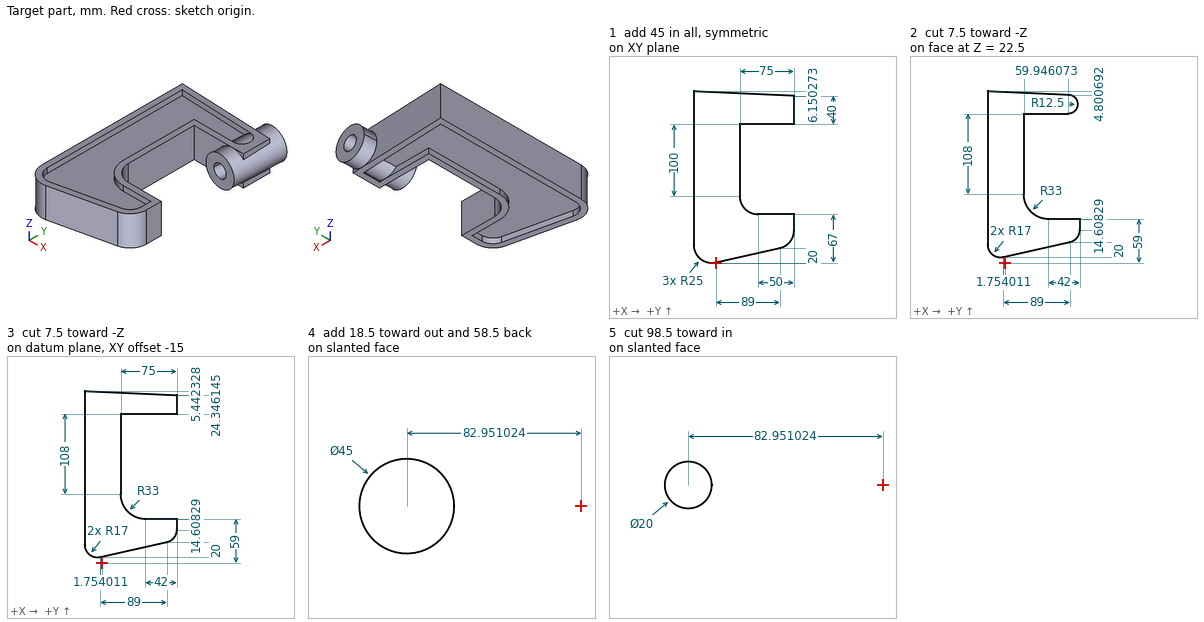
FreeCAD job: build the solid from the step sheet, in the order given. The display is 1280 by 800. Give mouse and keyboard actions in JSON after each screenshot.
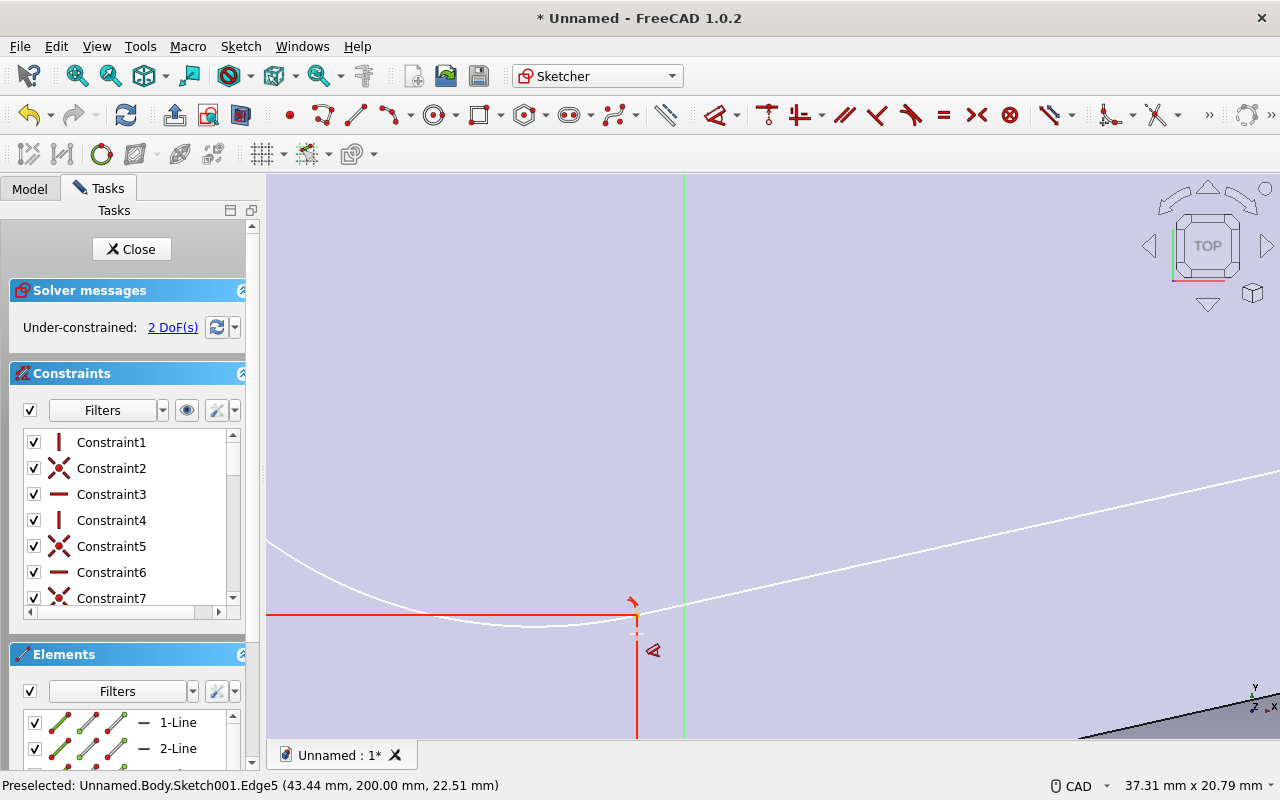
{"action": "left_click", "coordinate": [637, 615]}
{"action": "left_click", "coordinate": [660, 581]}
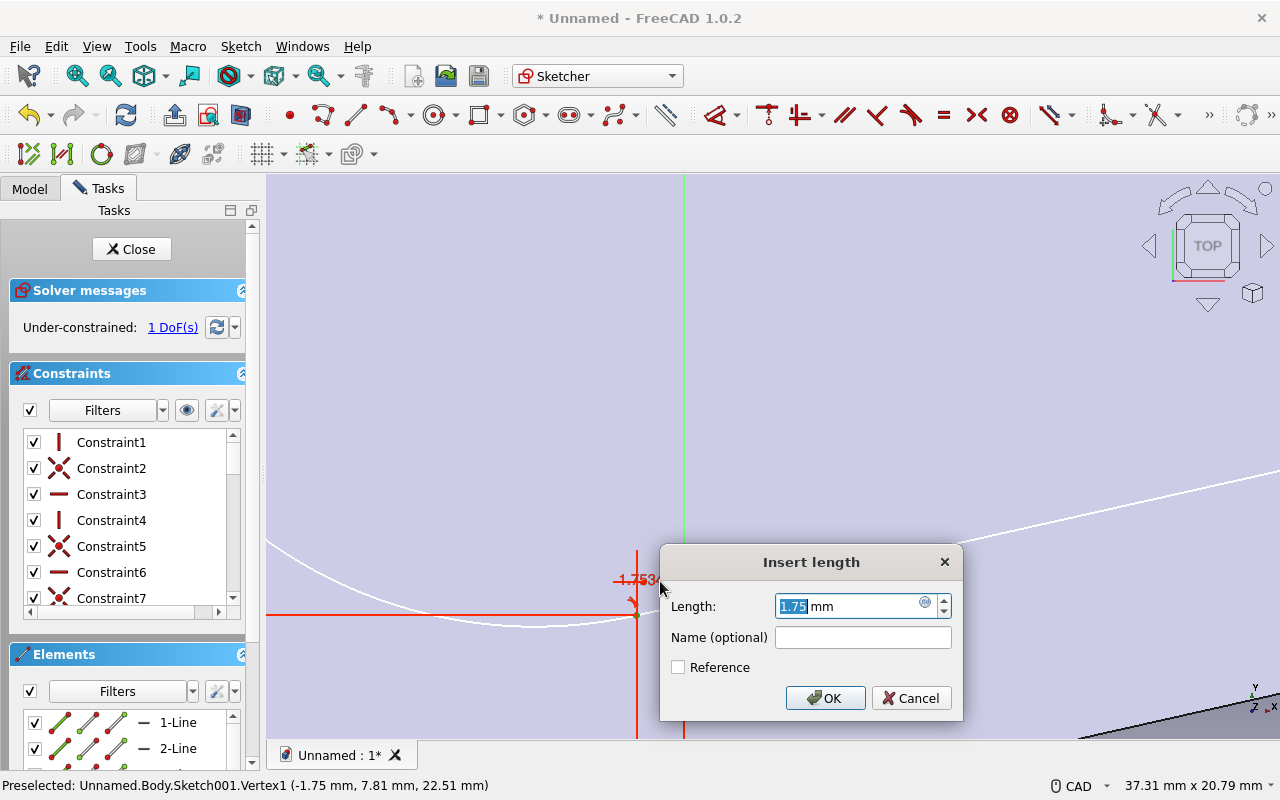
{"action": "type", "text": "1.754011"}
{"action": "key", "text": "Return"}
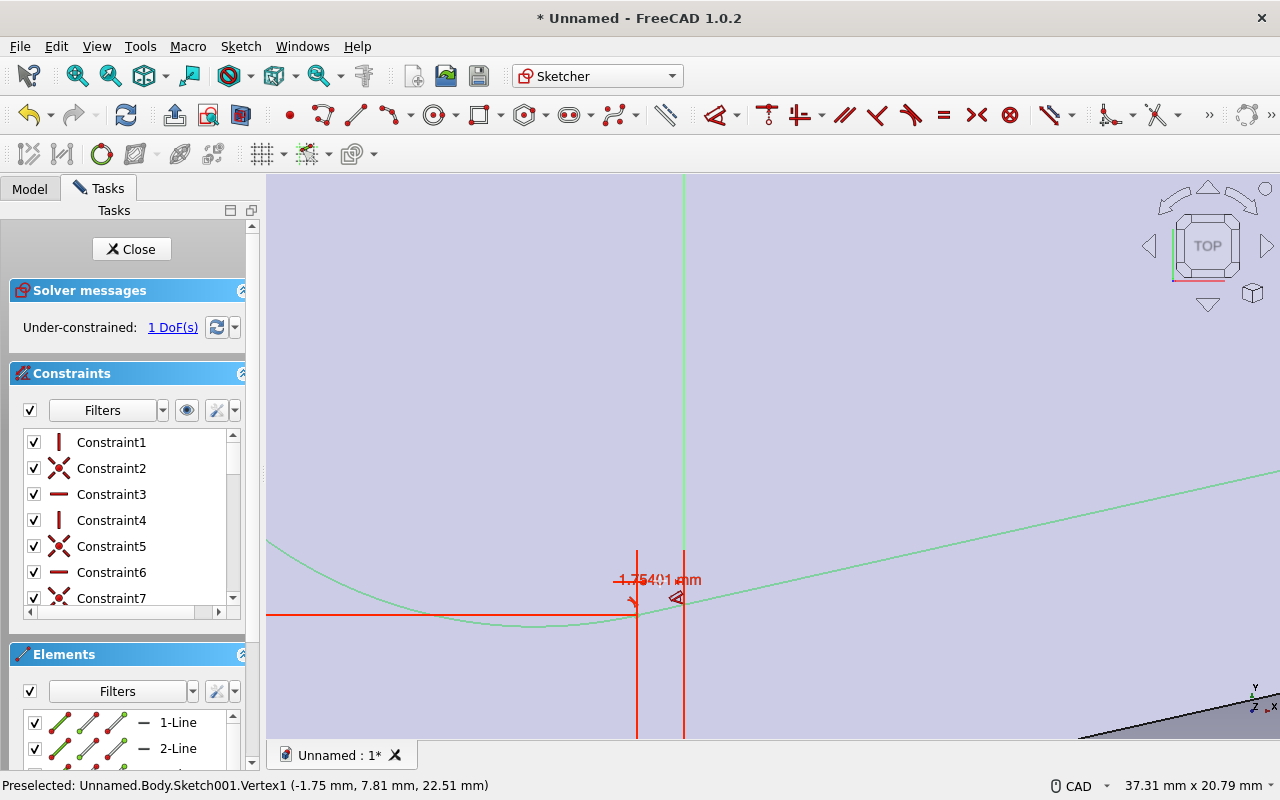
{"action": "scroll", "coordinate": [637, 635], "scroll_direction": "down", "scroll_amount": 14}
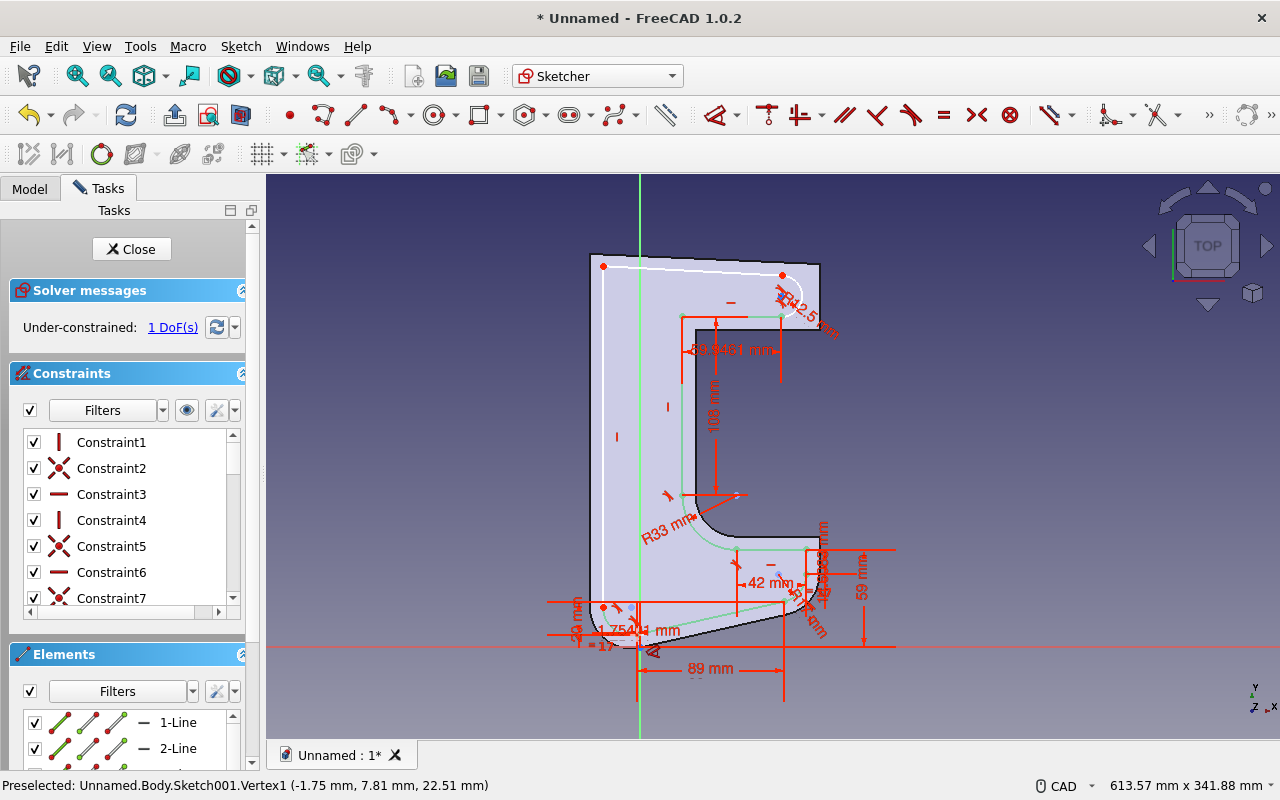
{"action": "scroll", "coordinate": [729, 273], "scroll_direction": "up", "scroll_amount": 9}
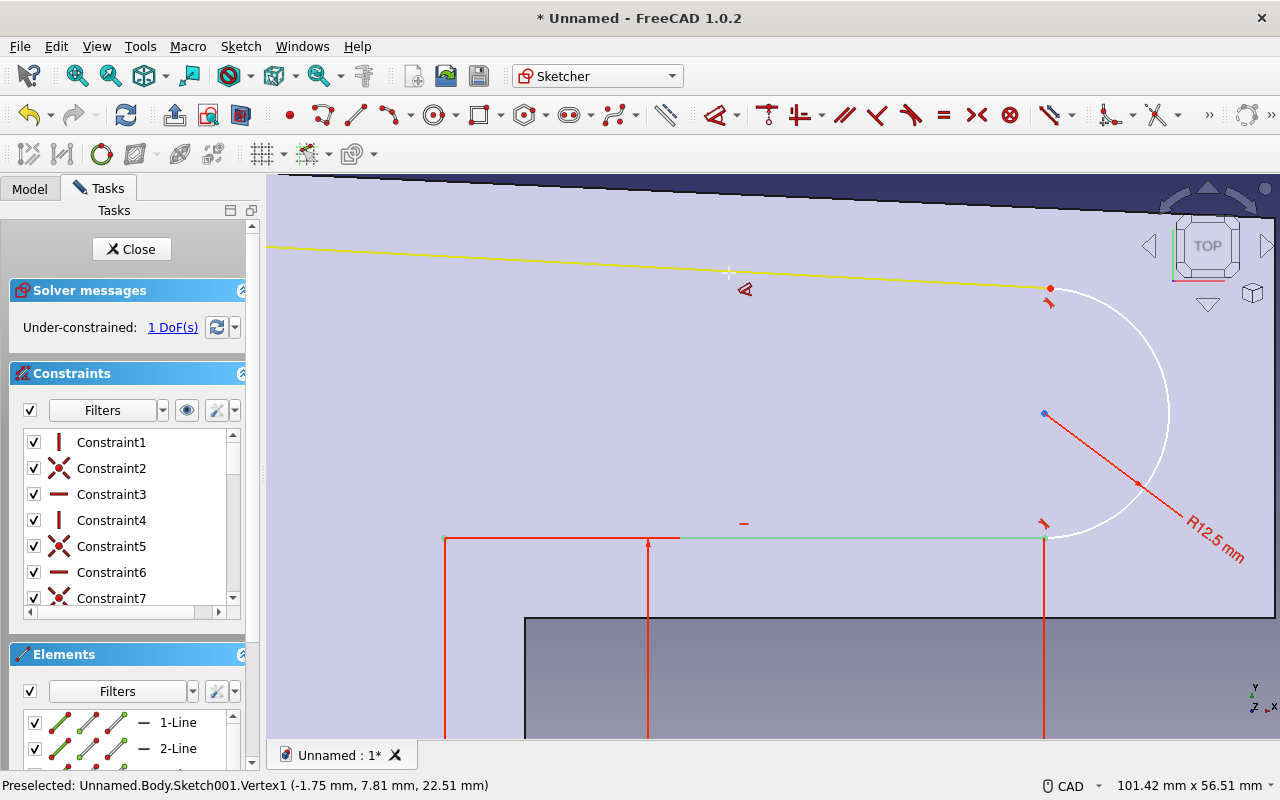
{"action": "left_click", "coordinate": [725, 271]}
{"action": "left_click", "coordinate": [1085, 260]}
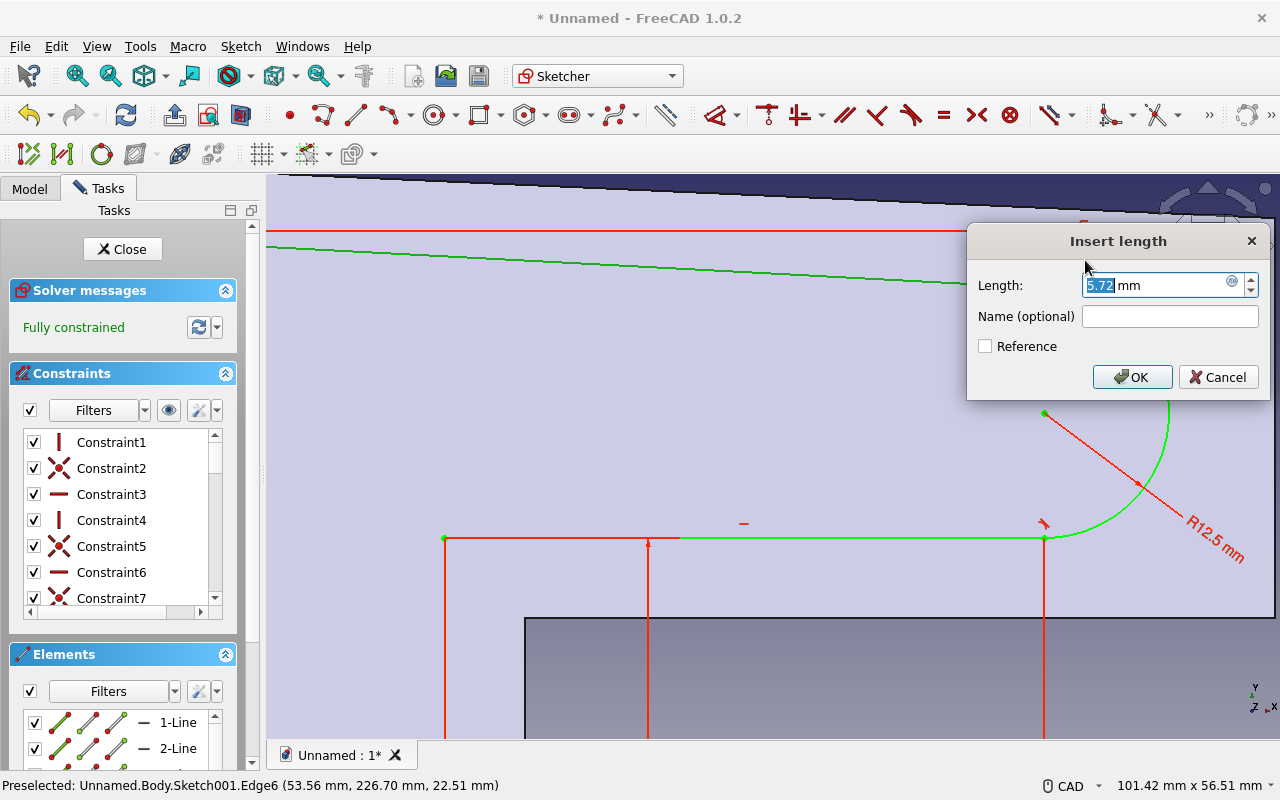
{"action": "type", "text": "4.800692"}
{"action": "key", "text": "Return"}
{"action": "key", "text": "Escape"}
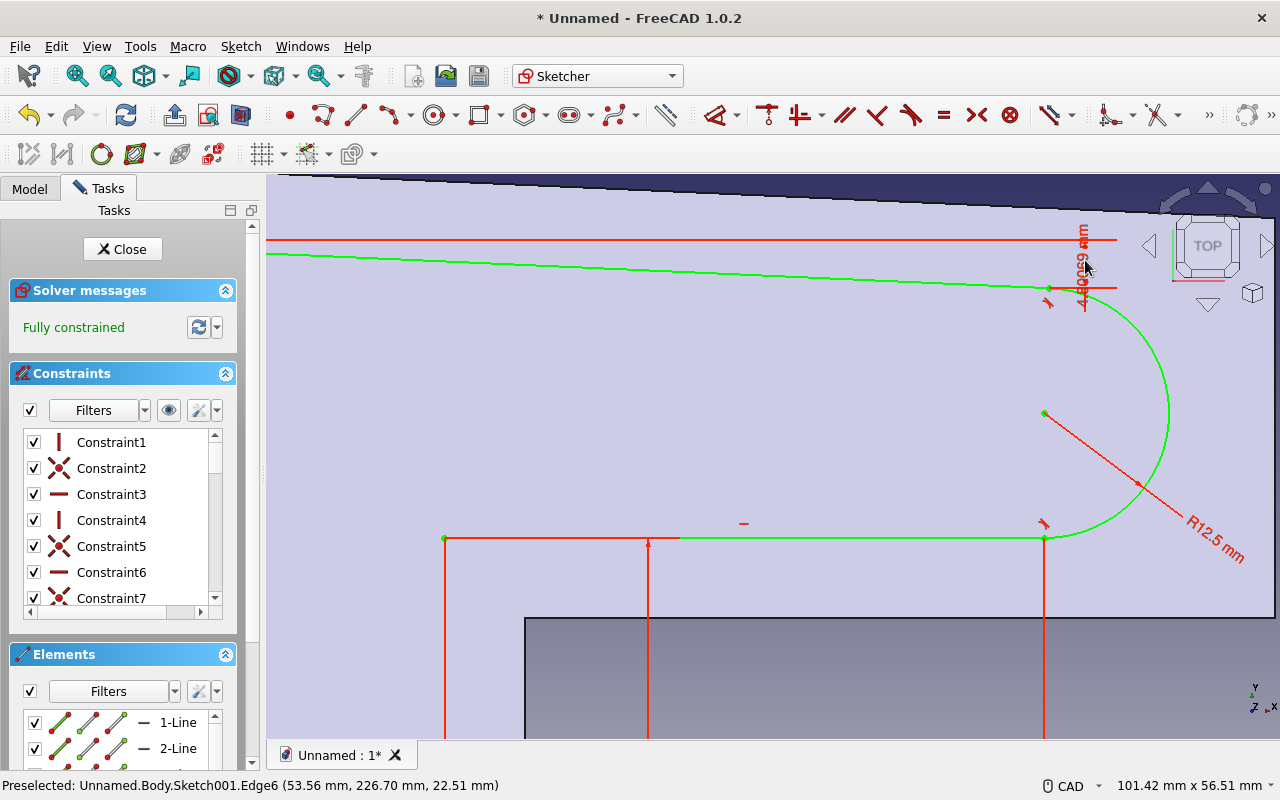
{"action": "left_click", "coordinate": [123, 249]}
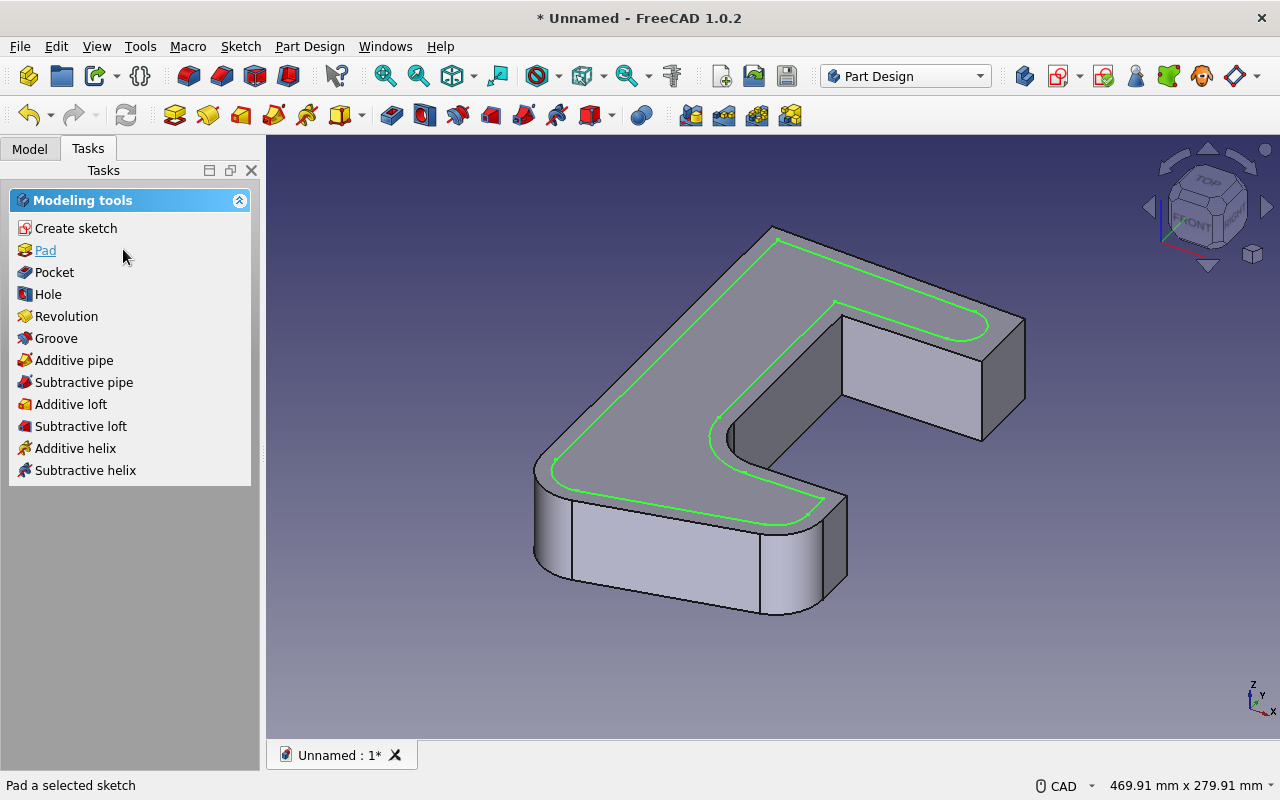
{"action": "left_click", "coordinate": [392, 116]}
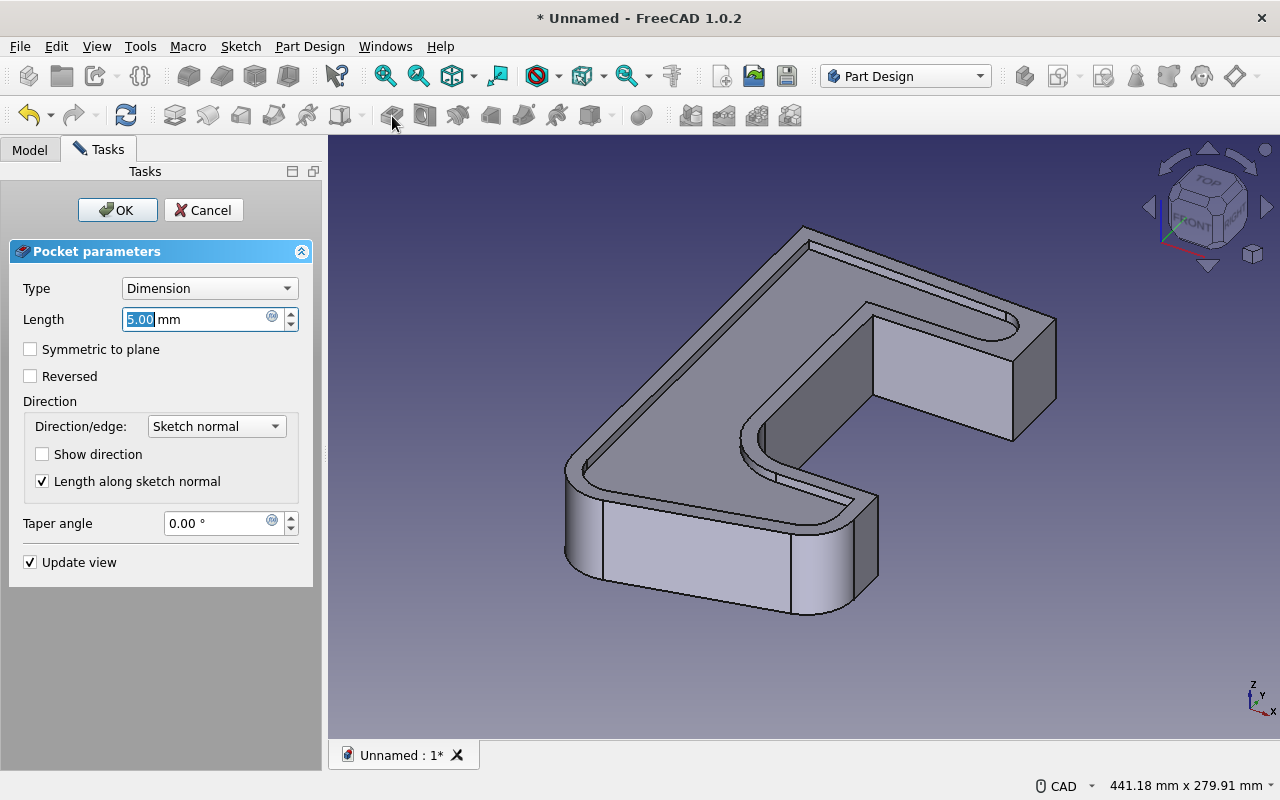
{"action": "type", "text": "7.5"}
{"action": "key", "text": "Tab"}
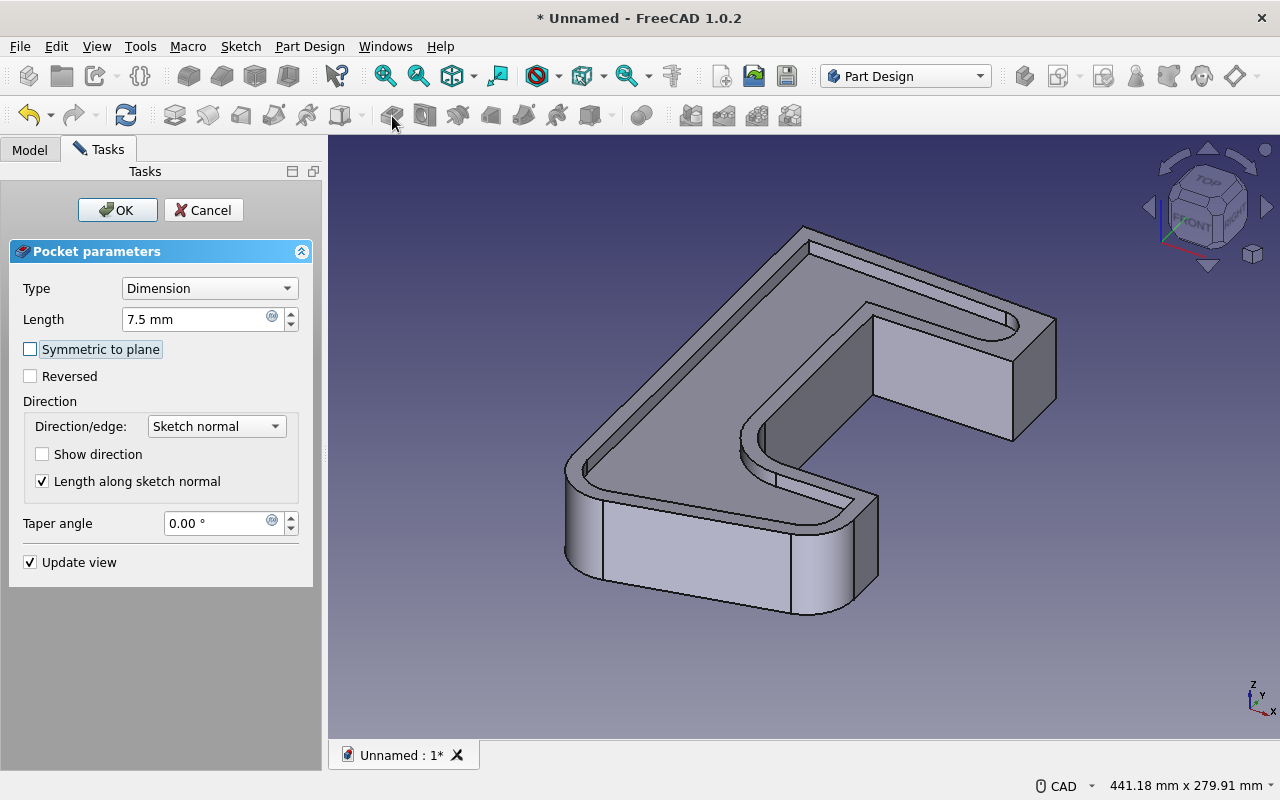
{"action": "left_click", "coordinate": [118, 210]}